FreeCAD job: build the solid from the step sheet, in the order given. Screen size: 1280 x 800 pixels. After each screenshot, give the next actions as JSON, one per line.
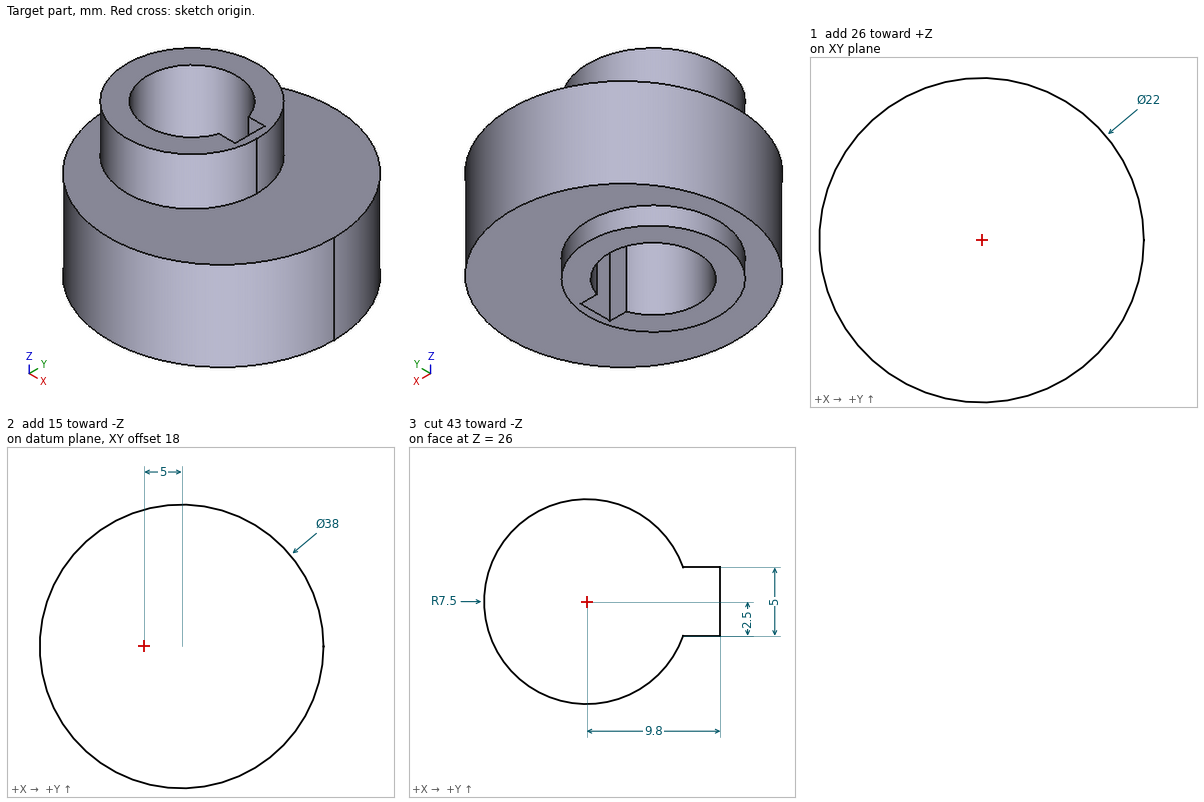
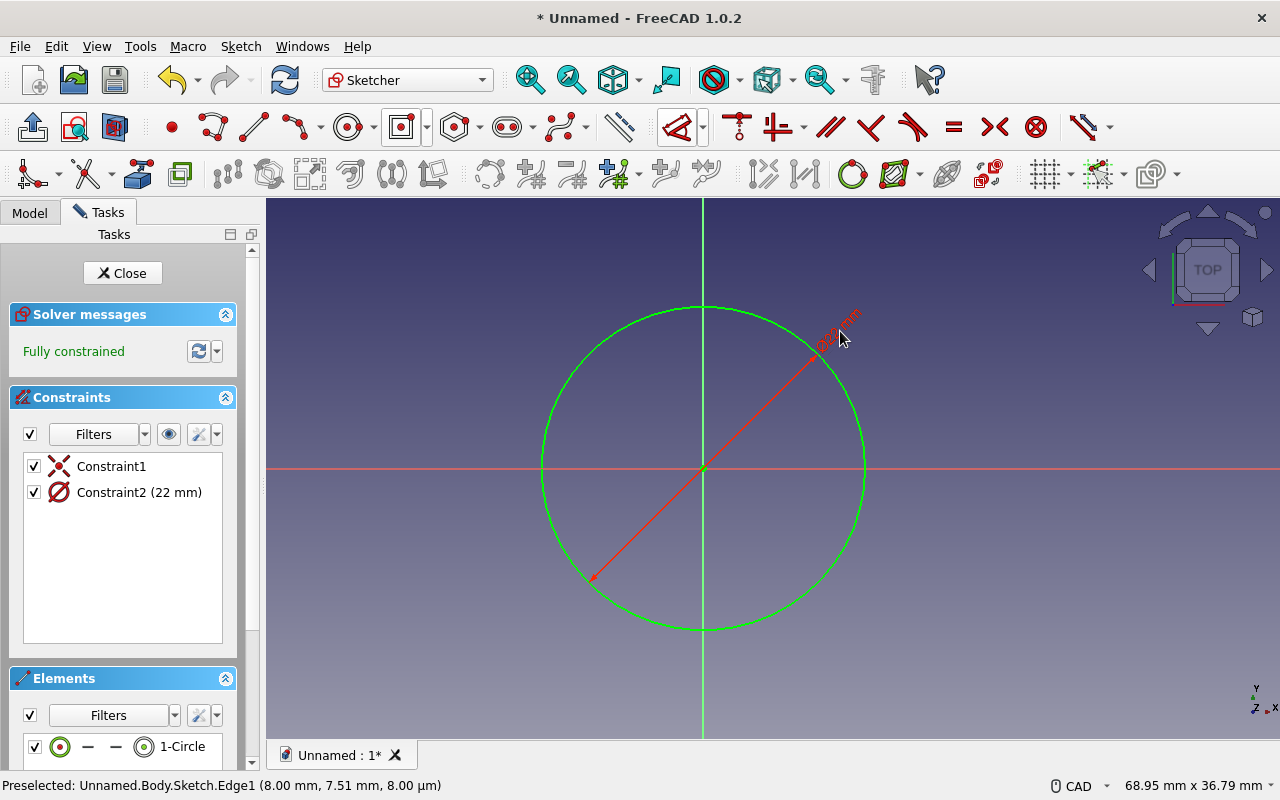
{"action": "left_click", "coordinate": [123, 273]}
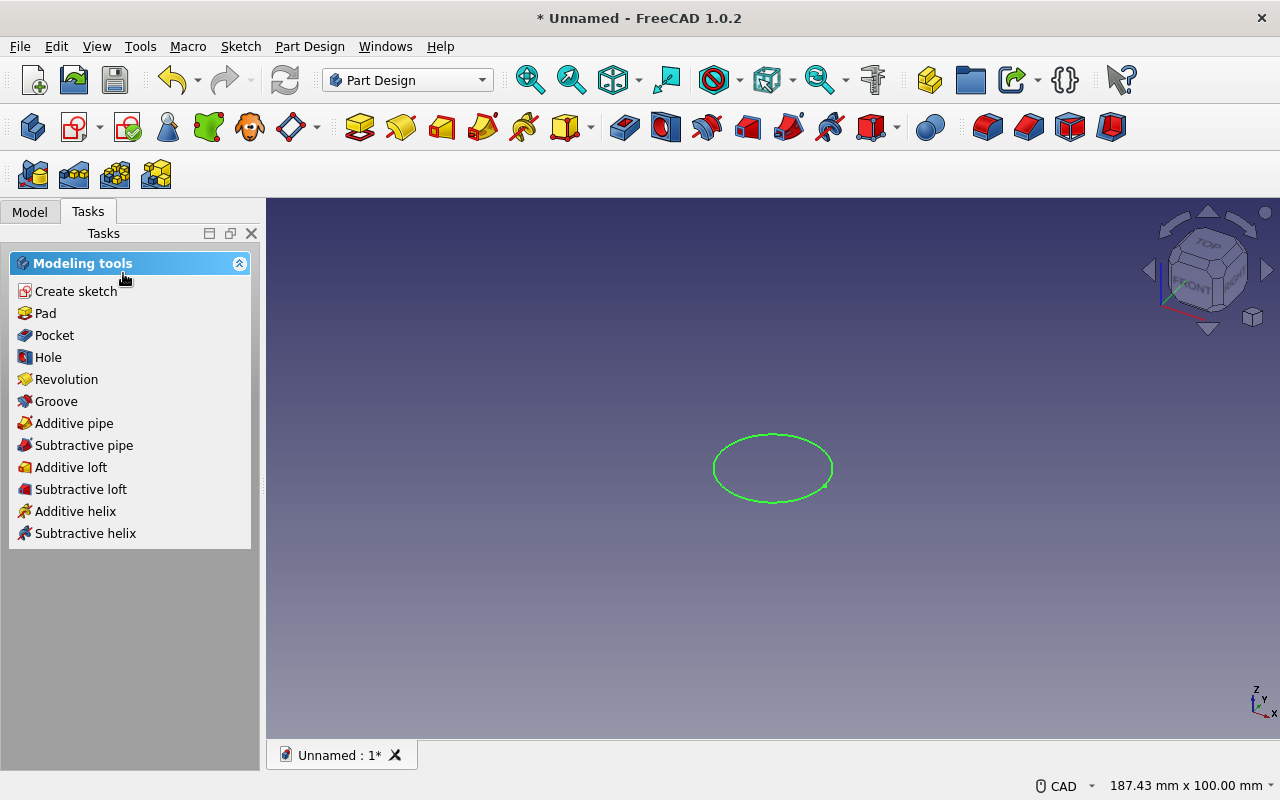
{"action": "left_click", "coordinate": [360, 128]}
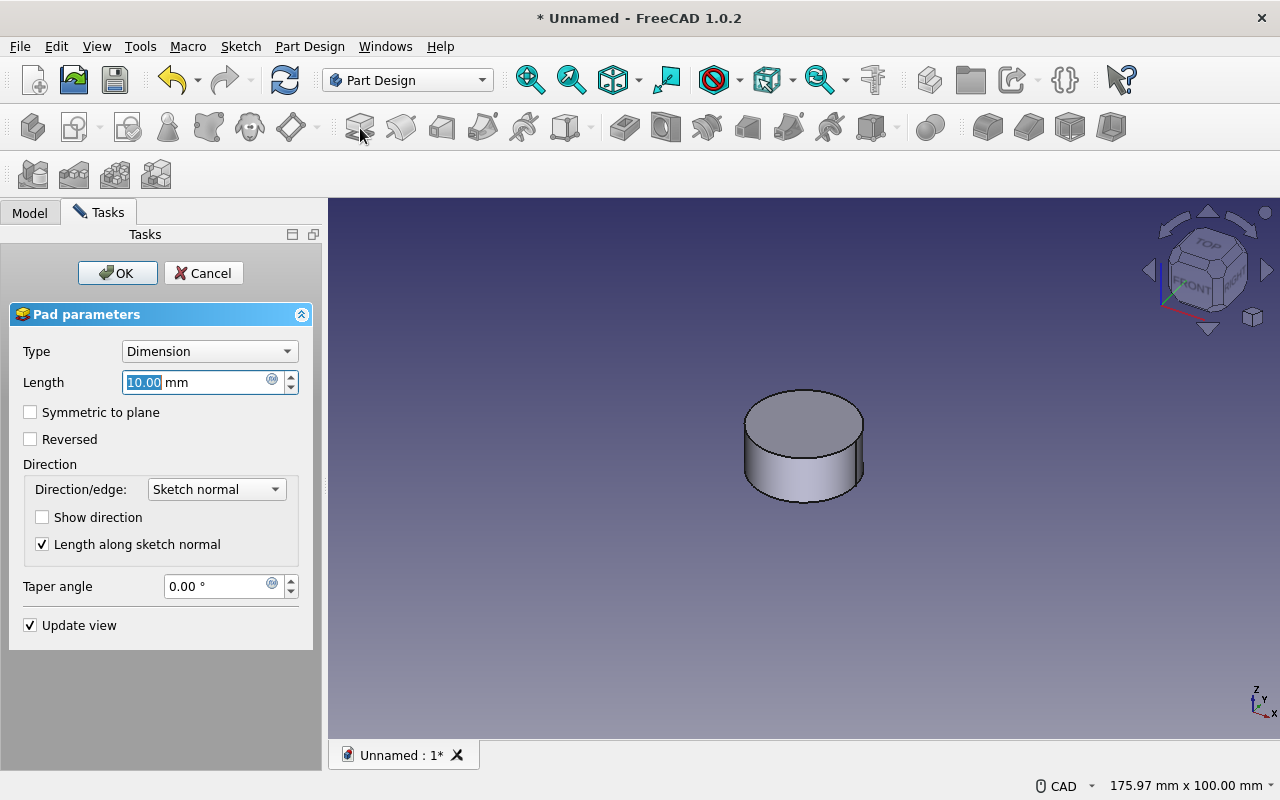
{"action": "type", "text": "26"}
{"action": "key", "text": "Tab"}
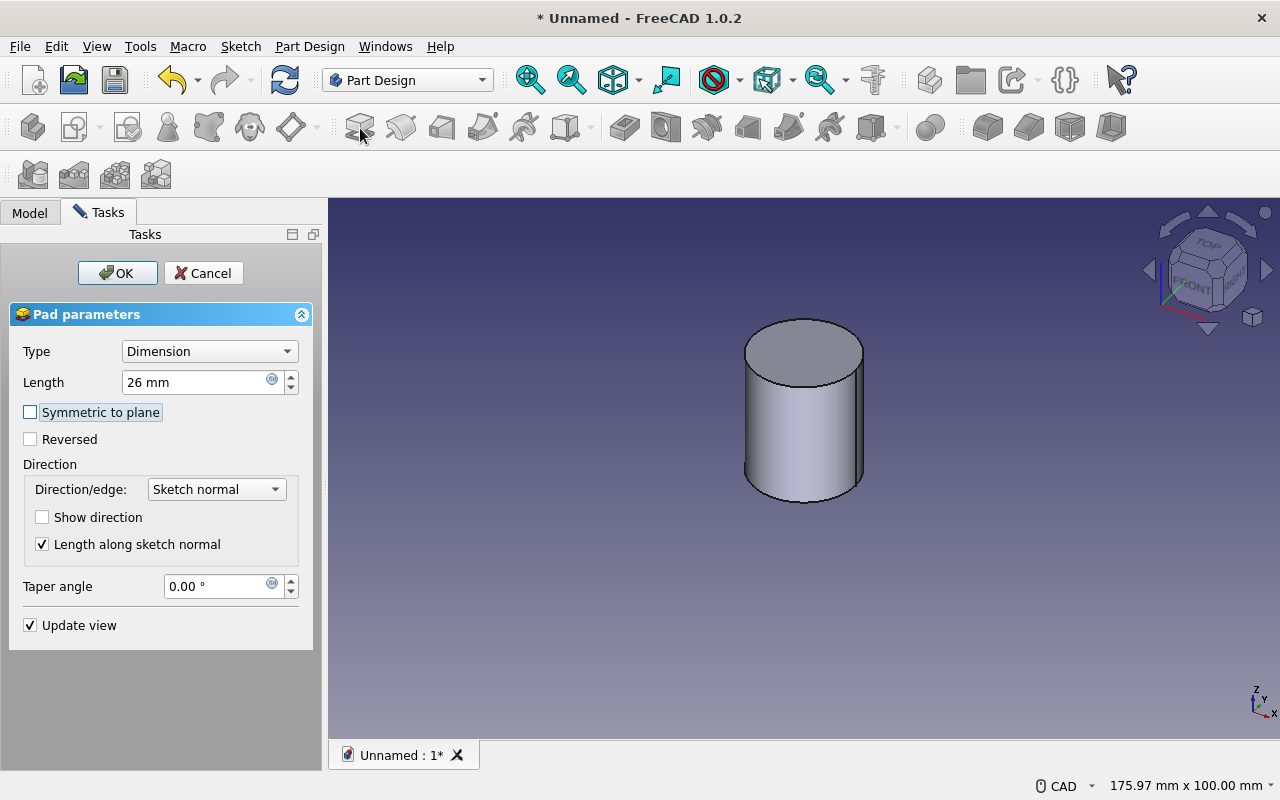
{"action": "left_click", "coordinate": [118, 273]}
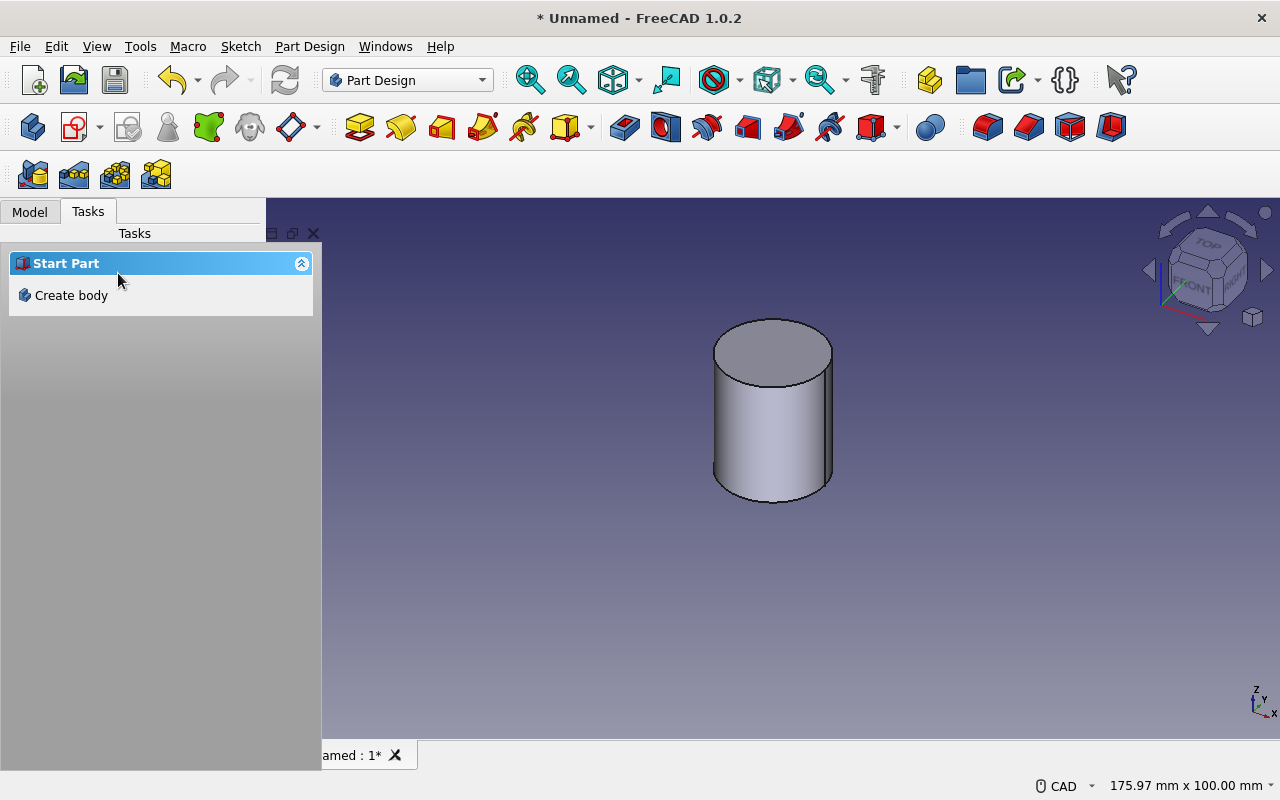
{"action": "left_click", "coordinate": [531, 80]}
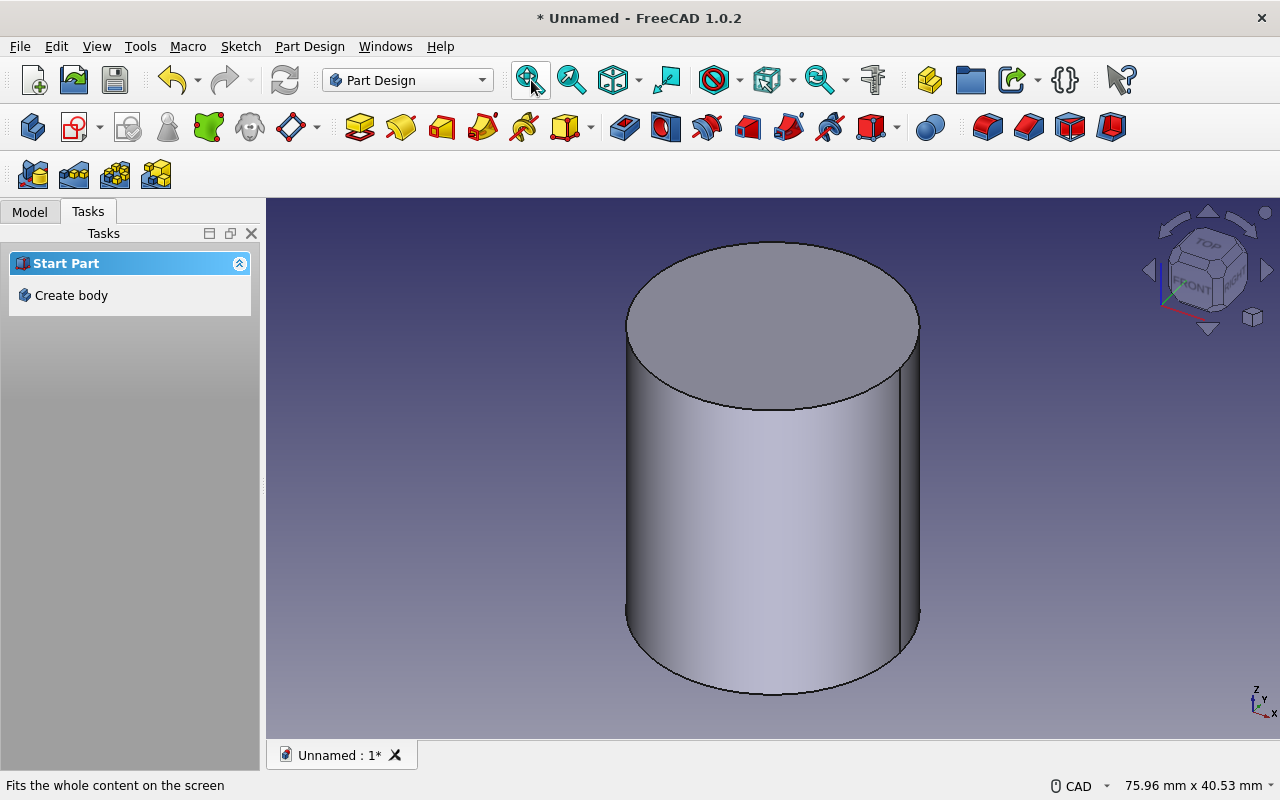
{"action": "left_click", "coordinate": [30, 212]}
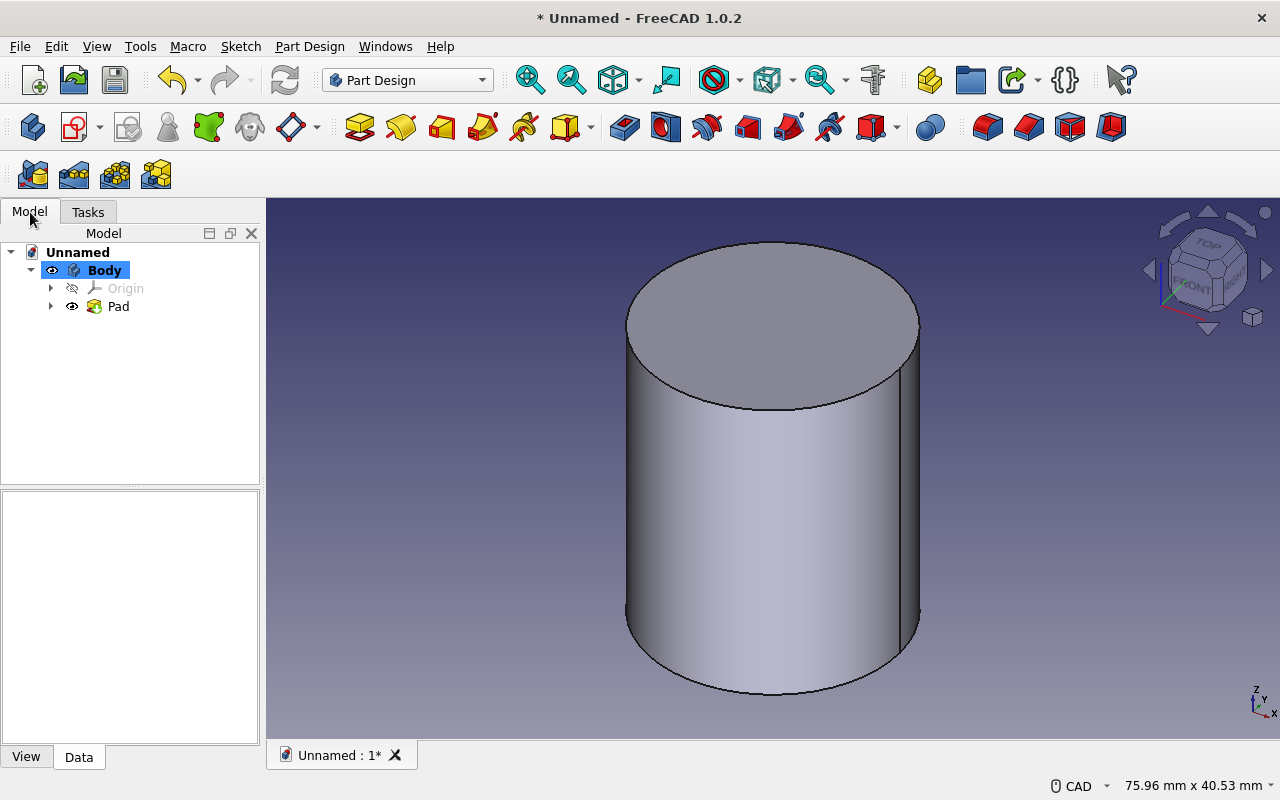
{"action": "left_click", "coordinate": [51, 288]}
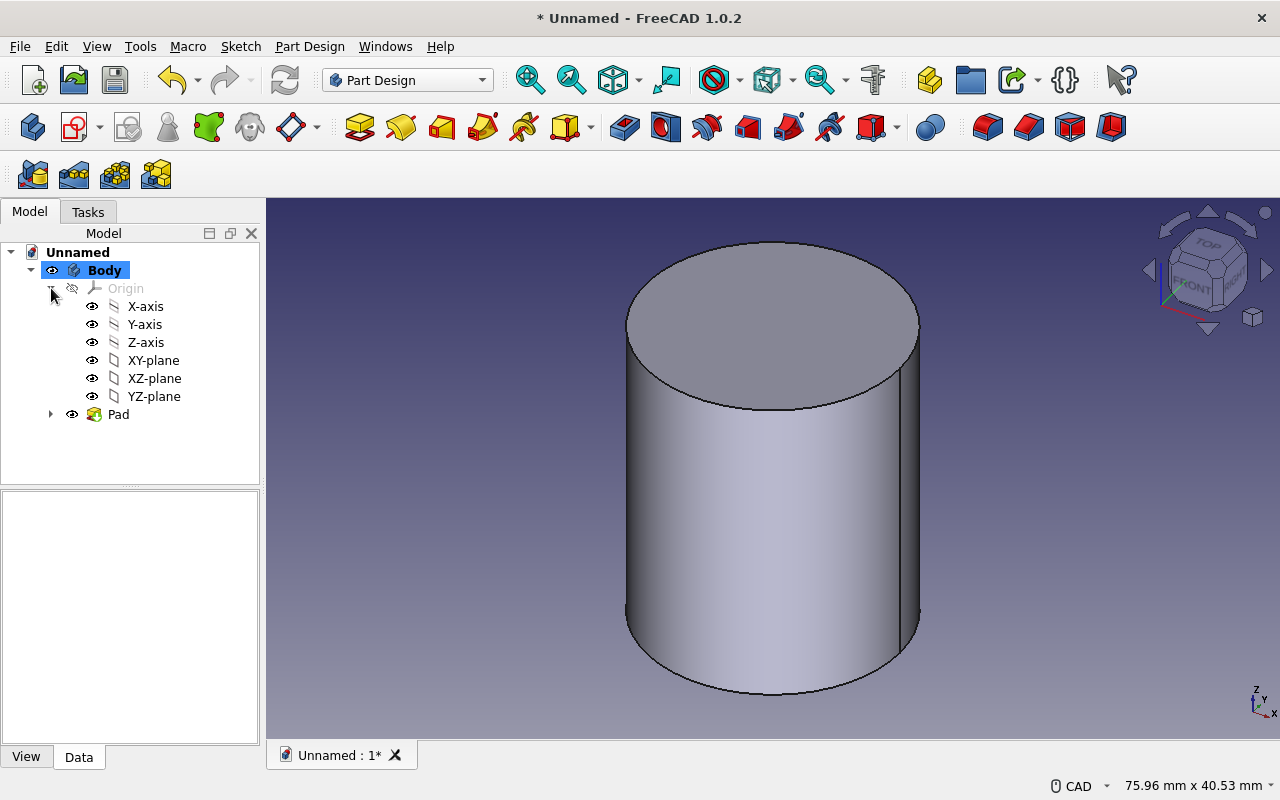
{"action": "left_click", "coordinate": [137, 360]}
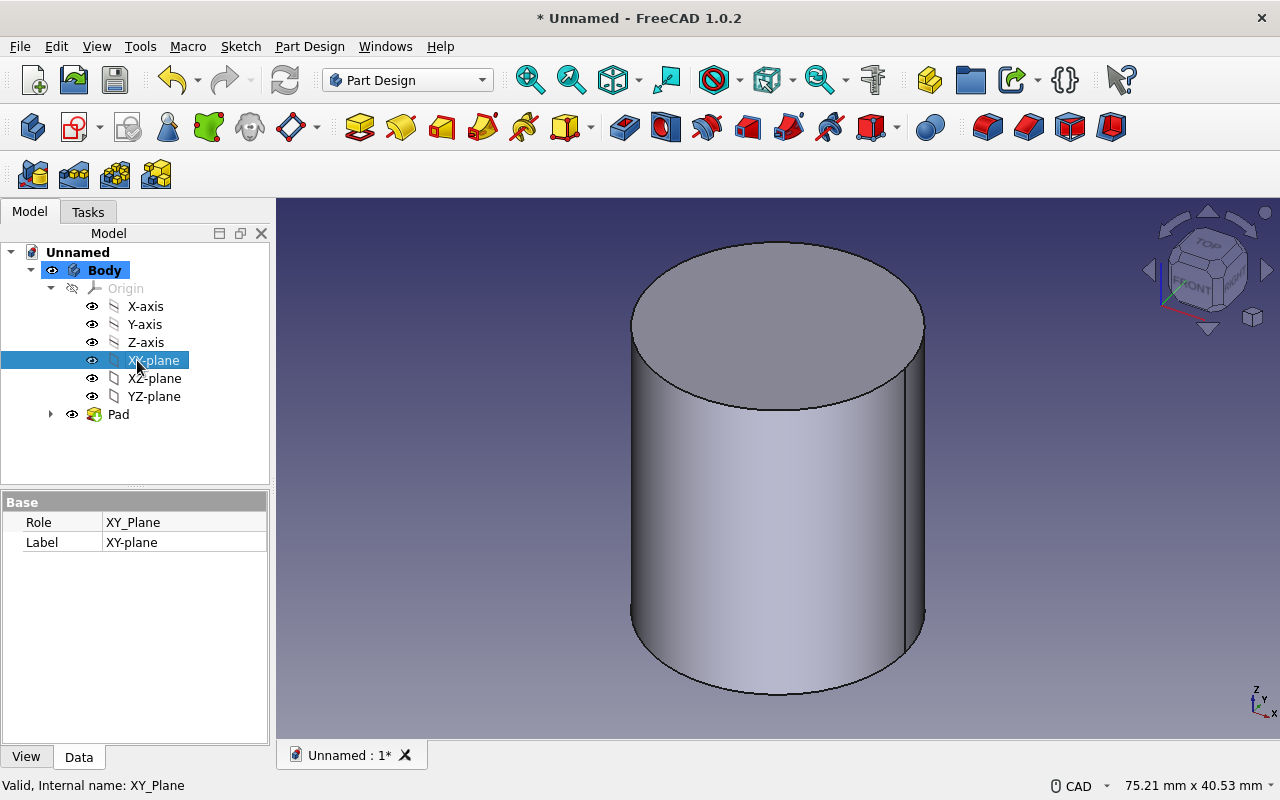
{"action": "left_click", "coordinate": [290, 128]}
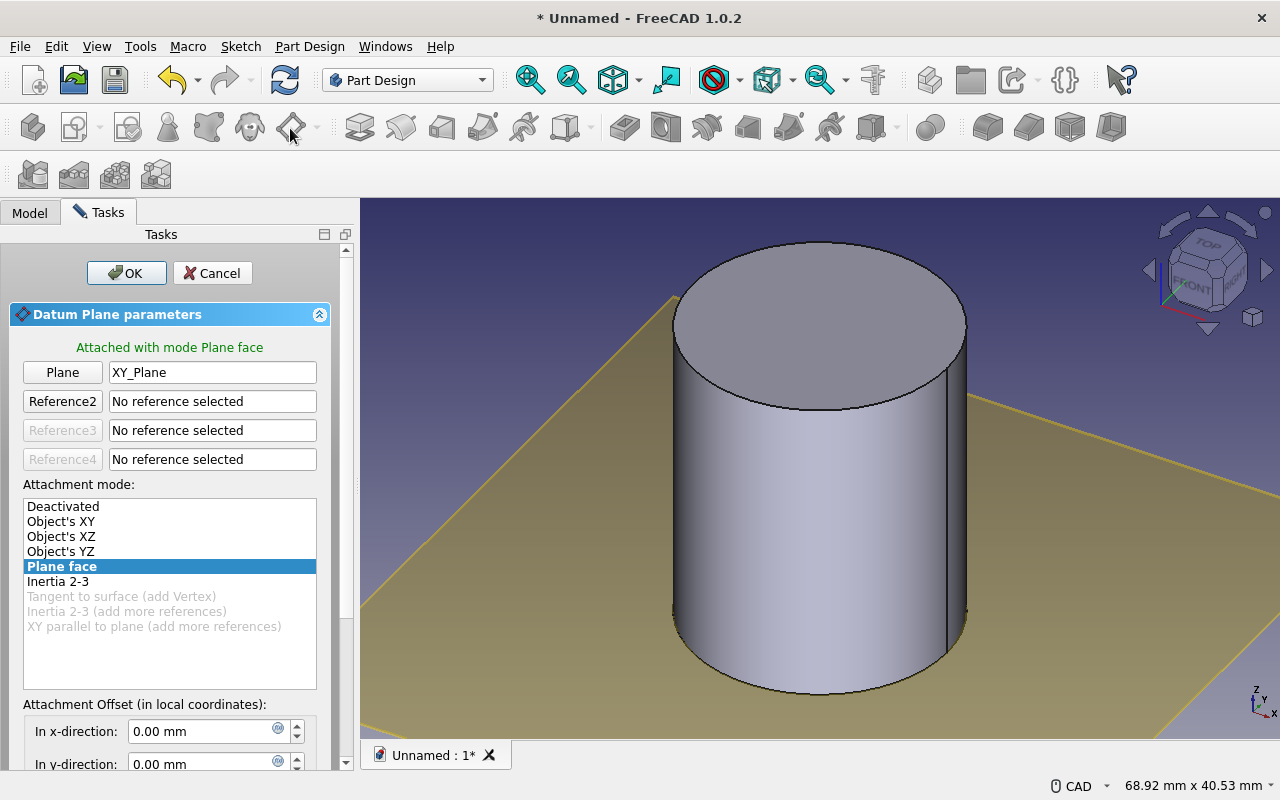
{"action": "scroll", "coordinate": [346, 507], "scroll_direction": "down", "scroll_amount": 2}